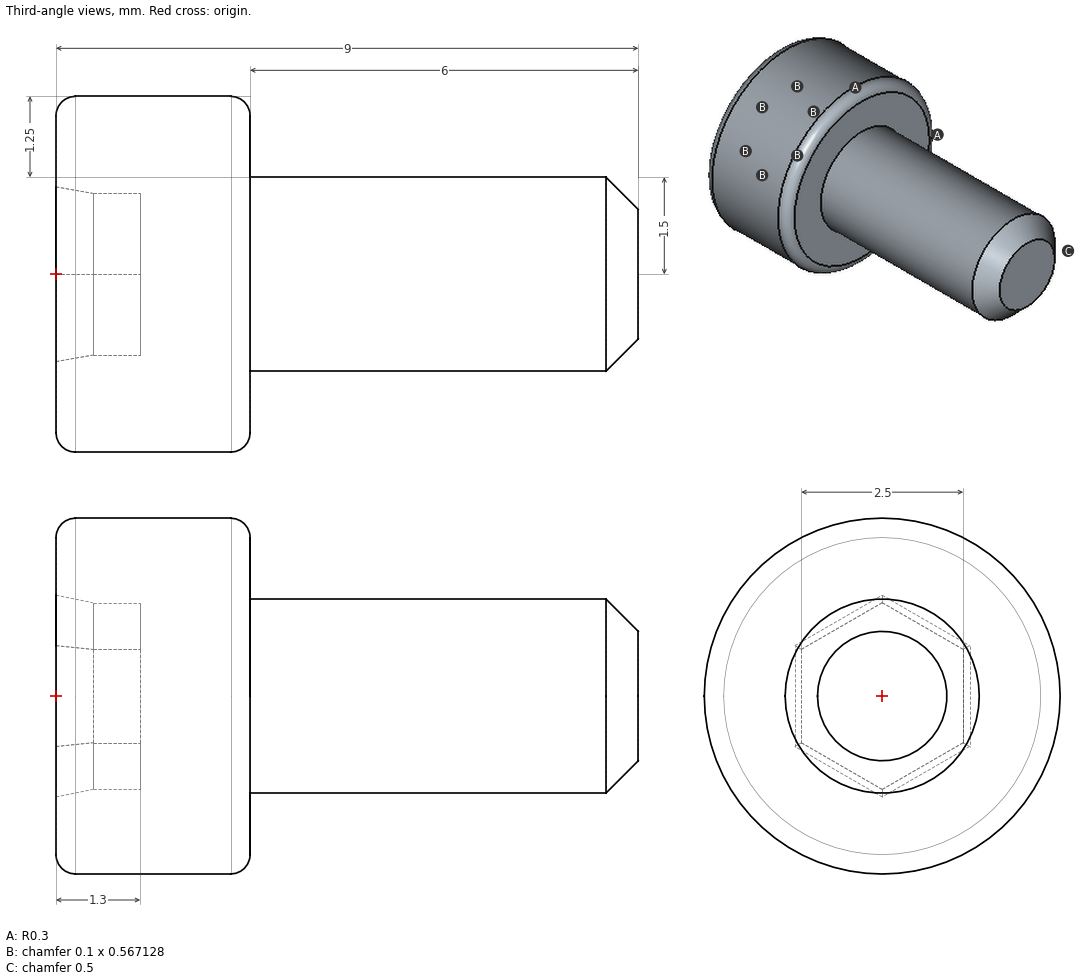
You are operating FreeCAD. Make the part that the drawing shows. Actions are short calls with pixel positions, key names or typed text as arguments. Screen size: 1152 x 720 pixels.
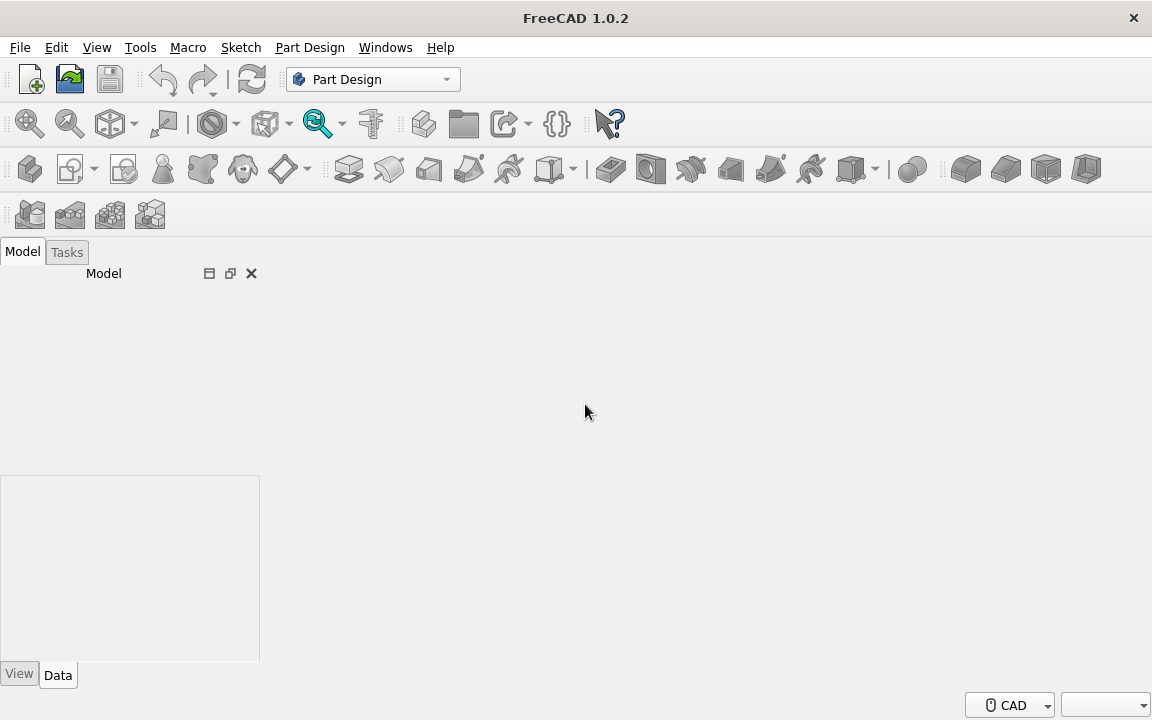
click(30, 80)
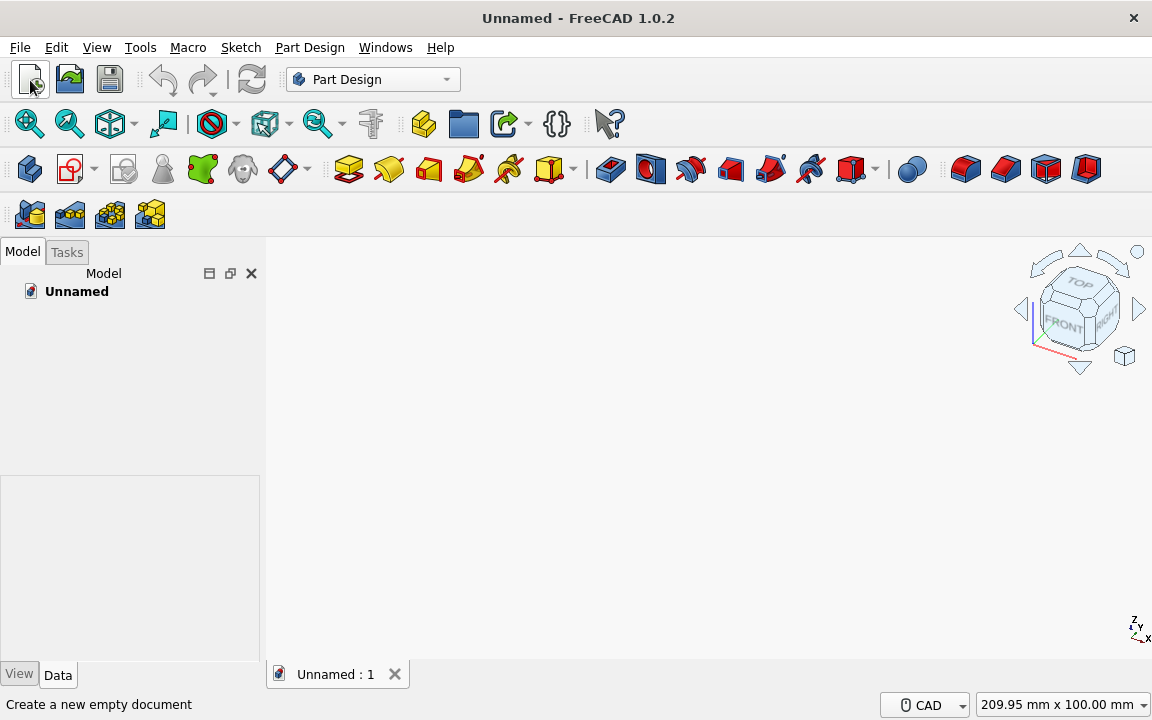
click(70, 170)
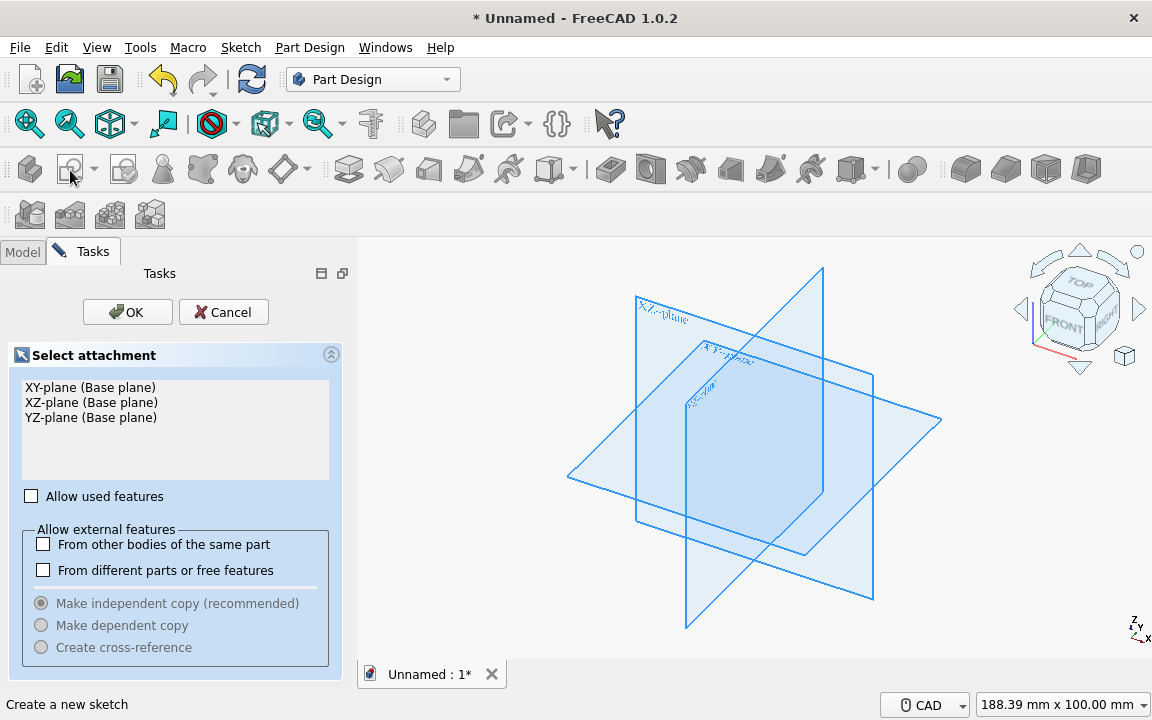
click(82, 388)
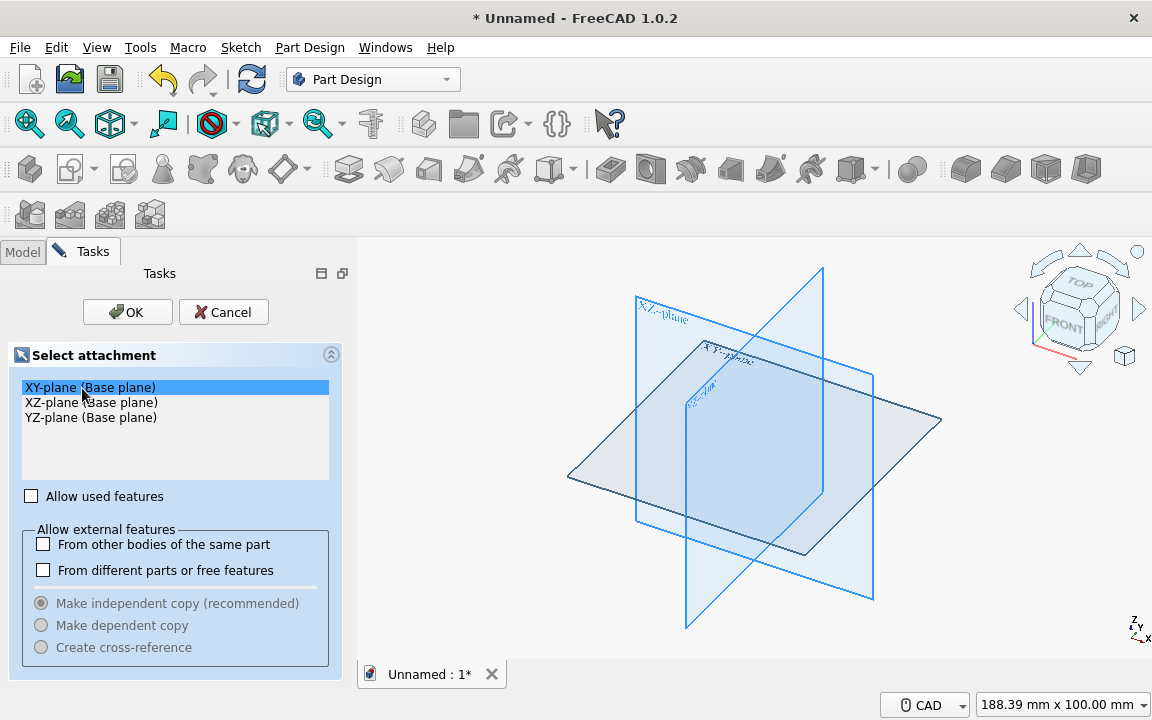
click(128, 312)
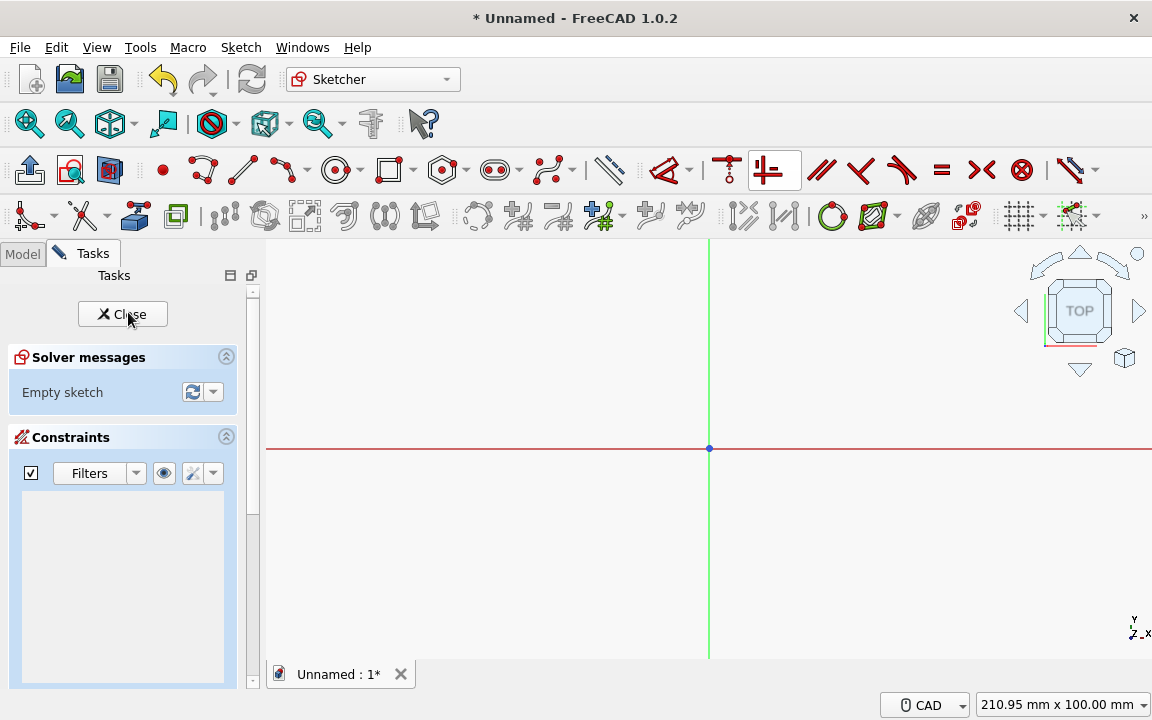
scroll(735, 443, up, 13)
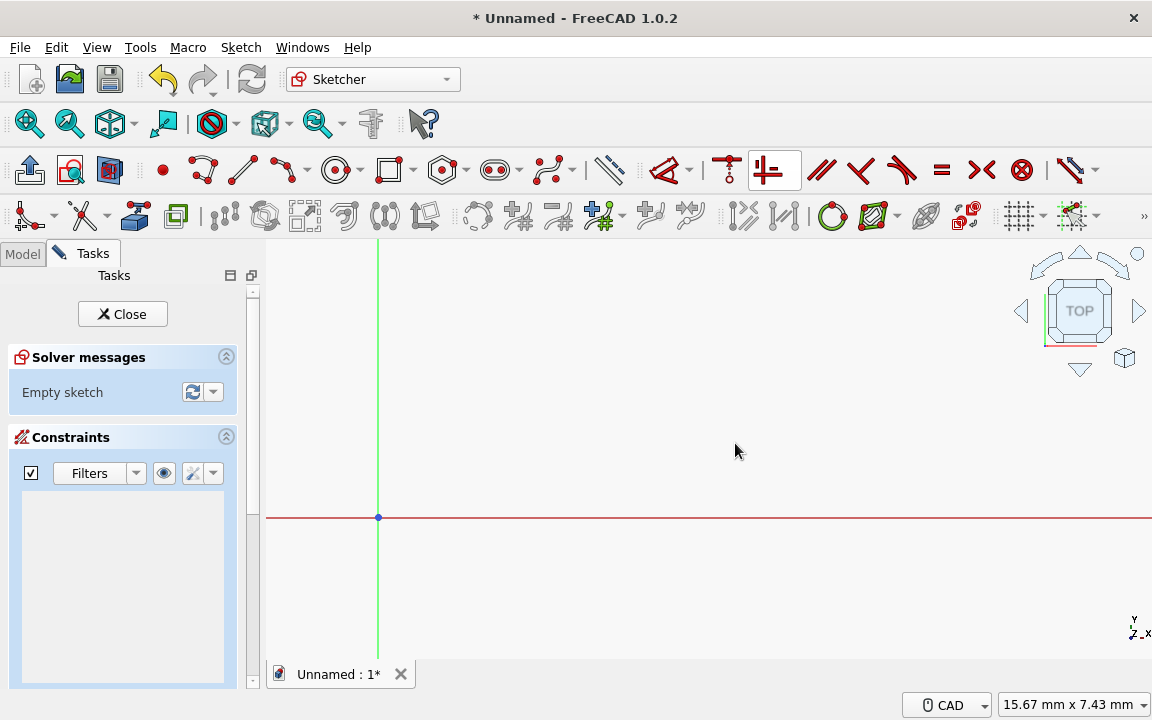
key(g)
key(m)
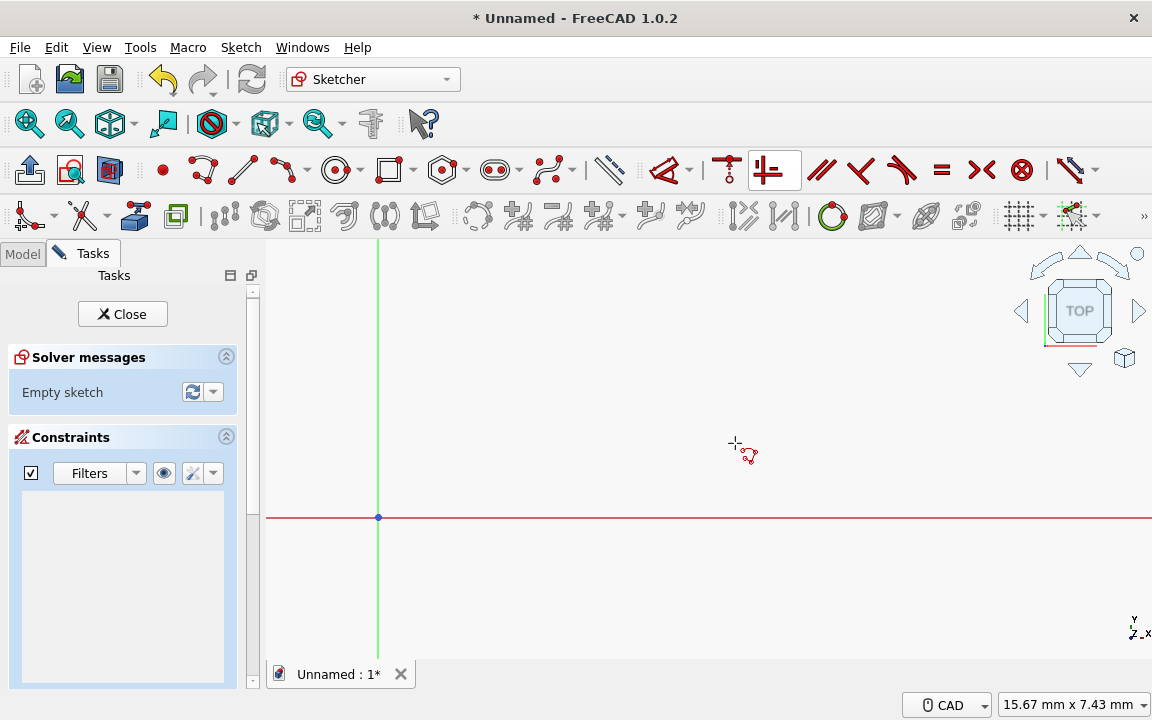
click(378, 518)
click(887, 509)
click(887, 433)
click(548, 433)
click(548, 362)
click(387, 362)
click(378, 518)
key(Escape)
key(Escape)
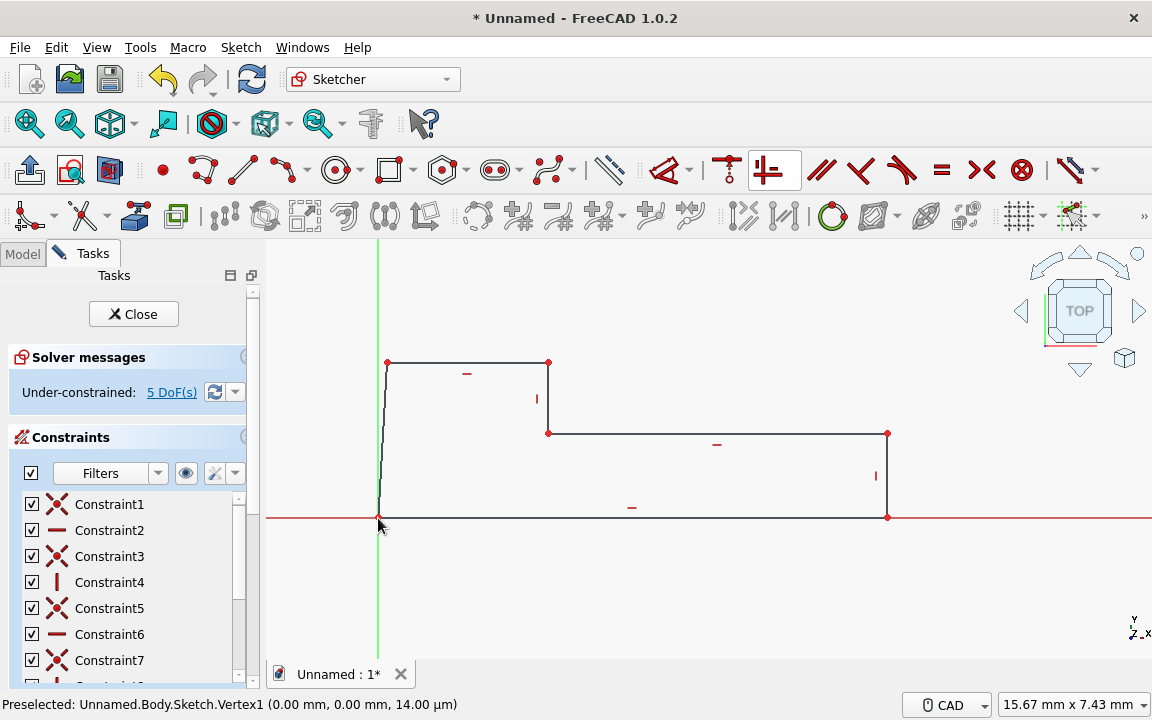
click(381, 471)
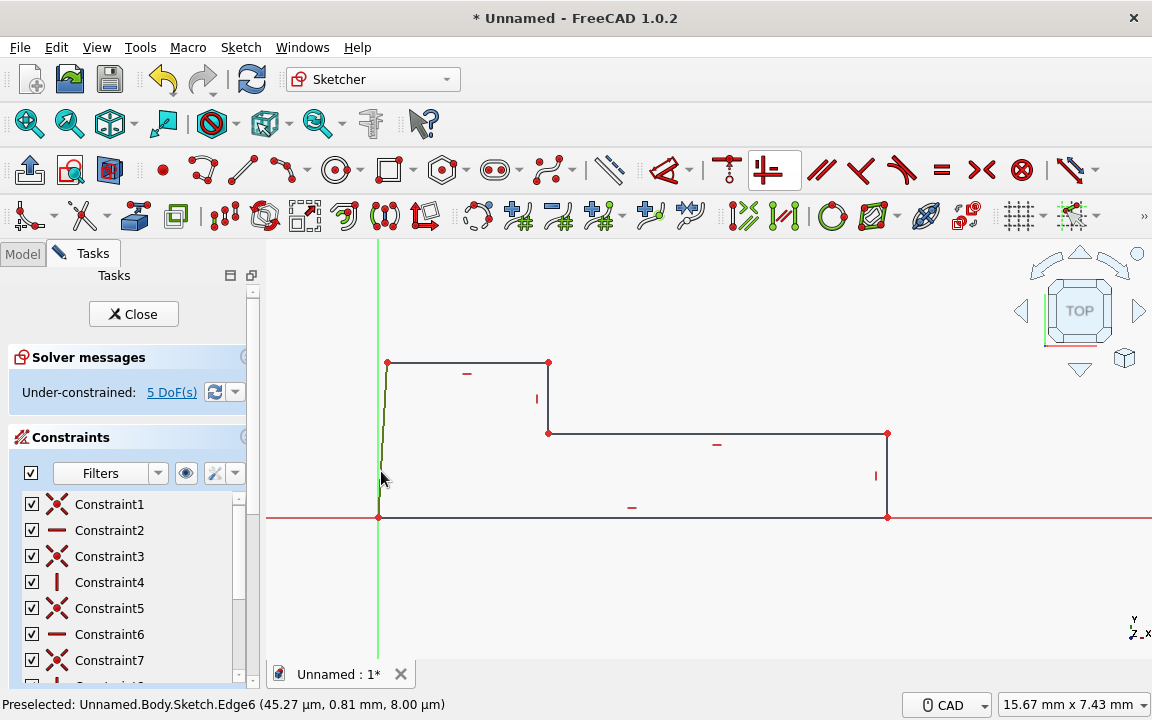
click(796, 170)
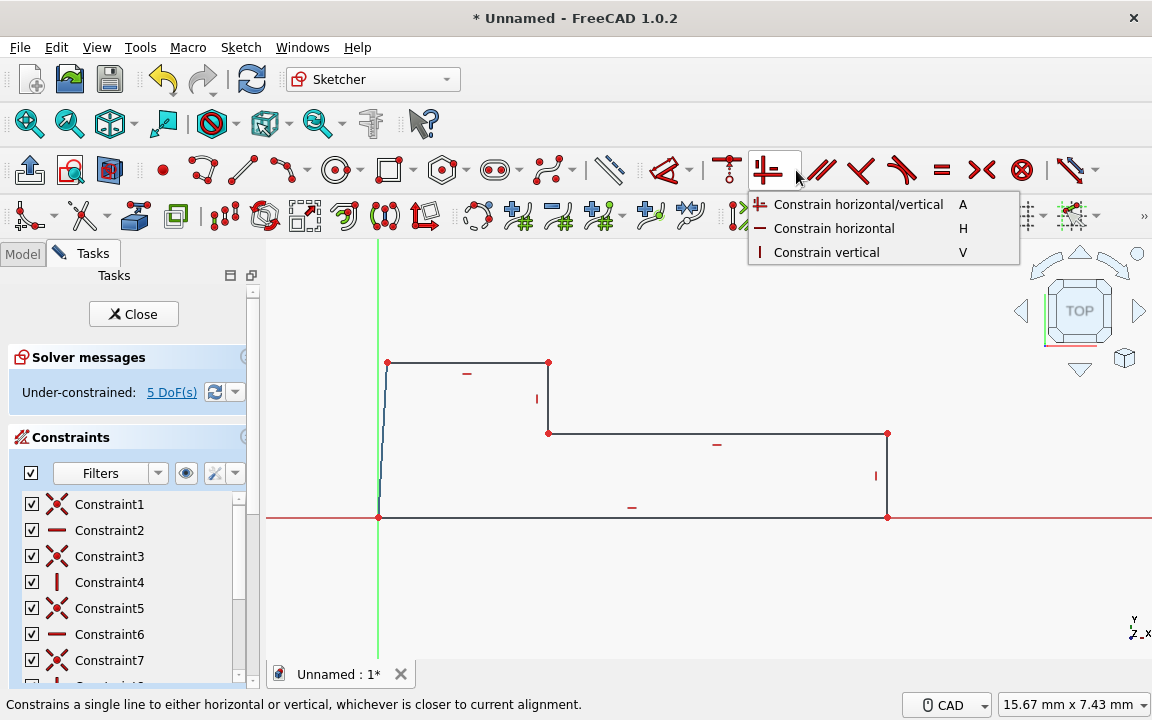
click(884, 252)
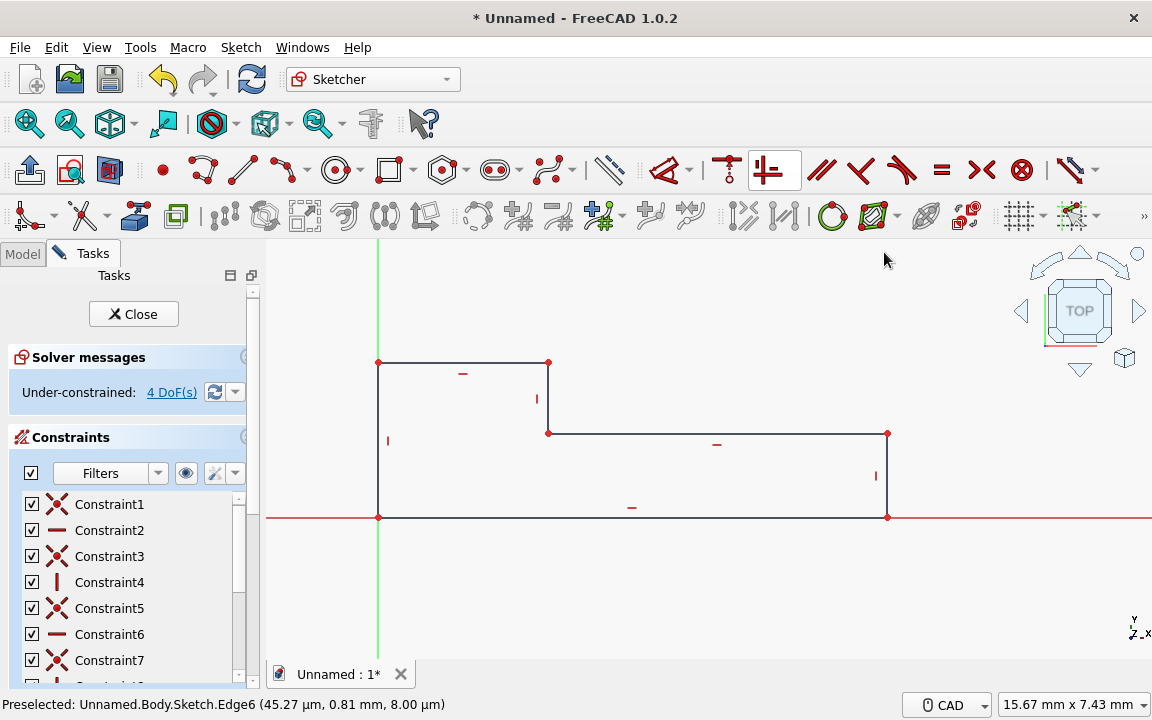
key(d)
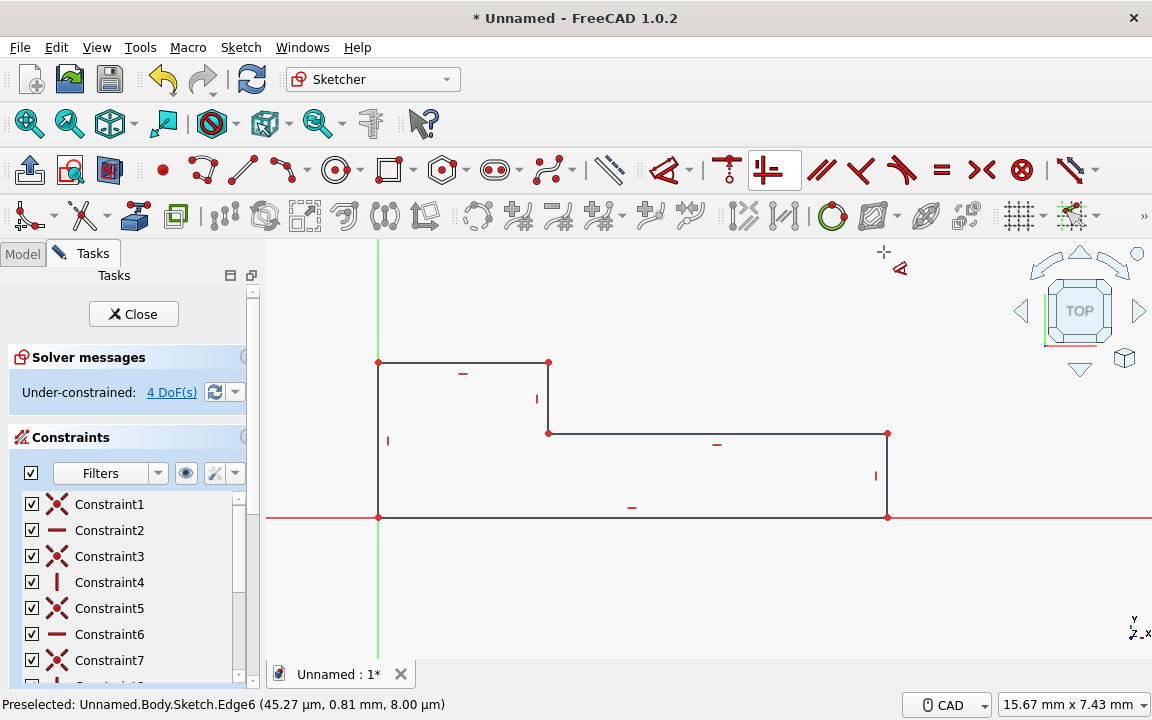
click(531, 518)
click(633, 552)